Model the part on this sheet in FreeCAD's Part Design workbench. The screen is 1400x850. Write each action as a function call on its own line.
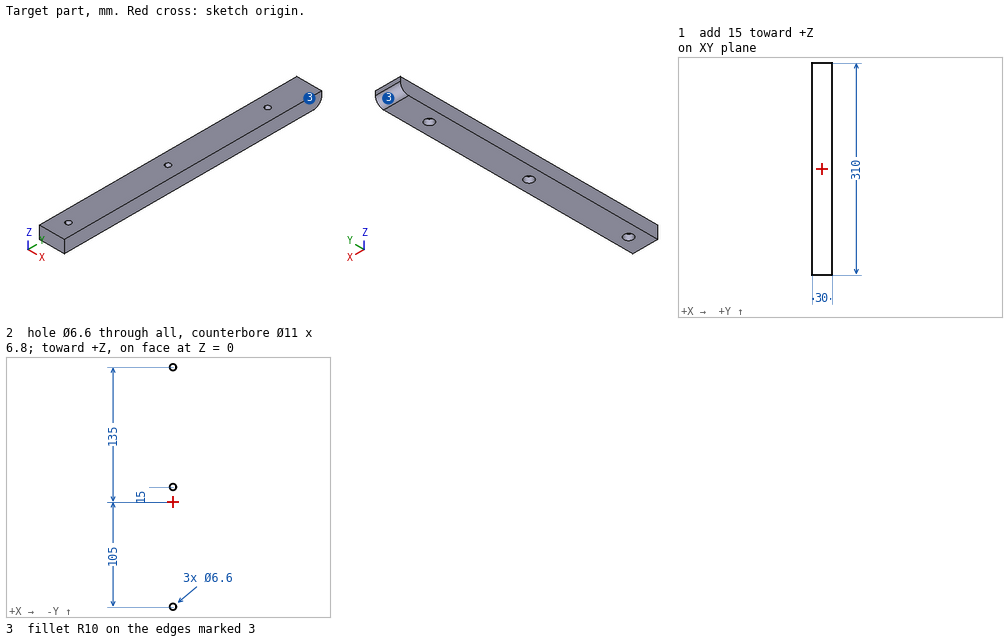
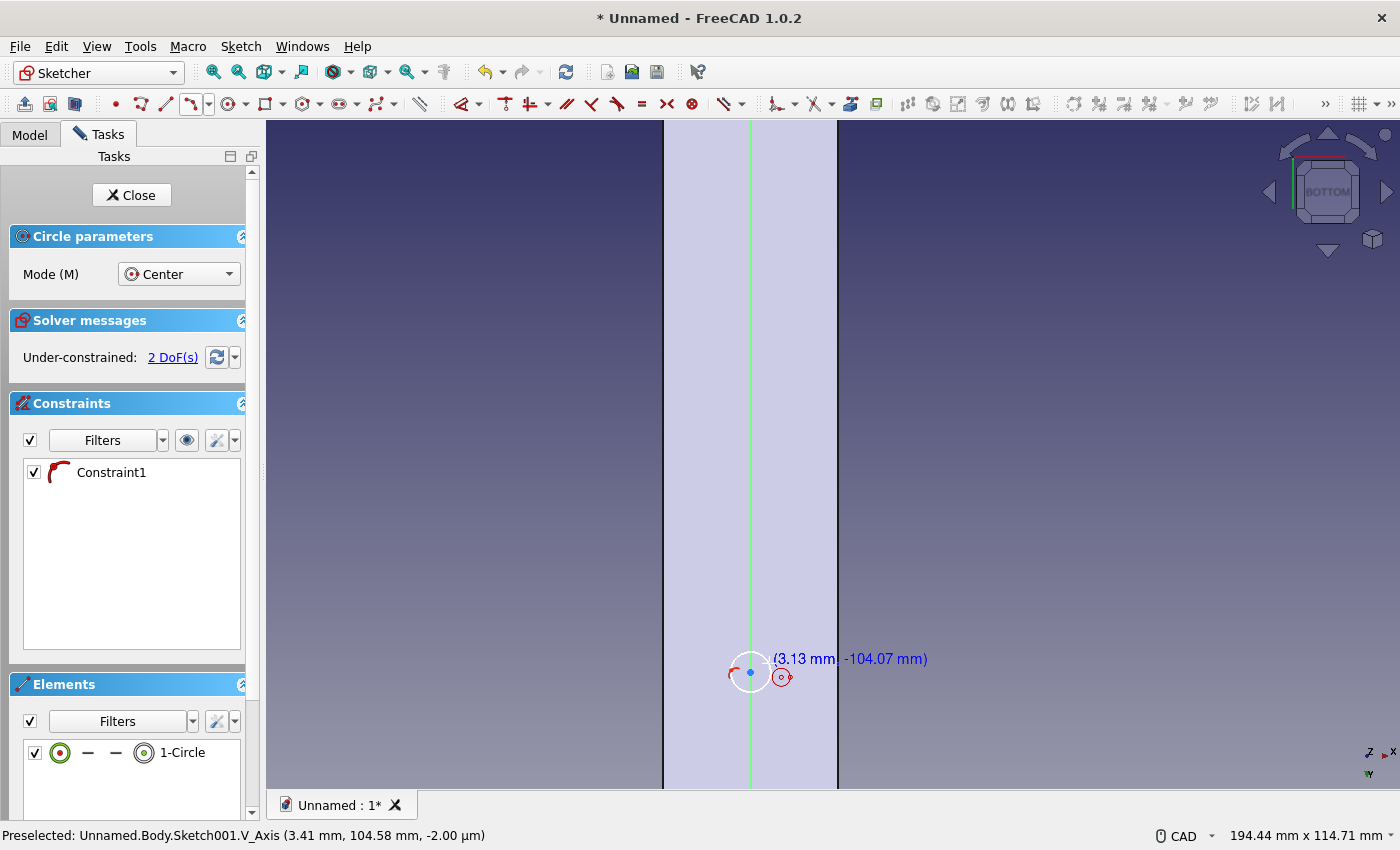
scroll(770, 664, down, 6)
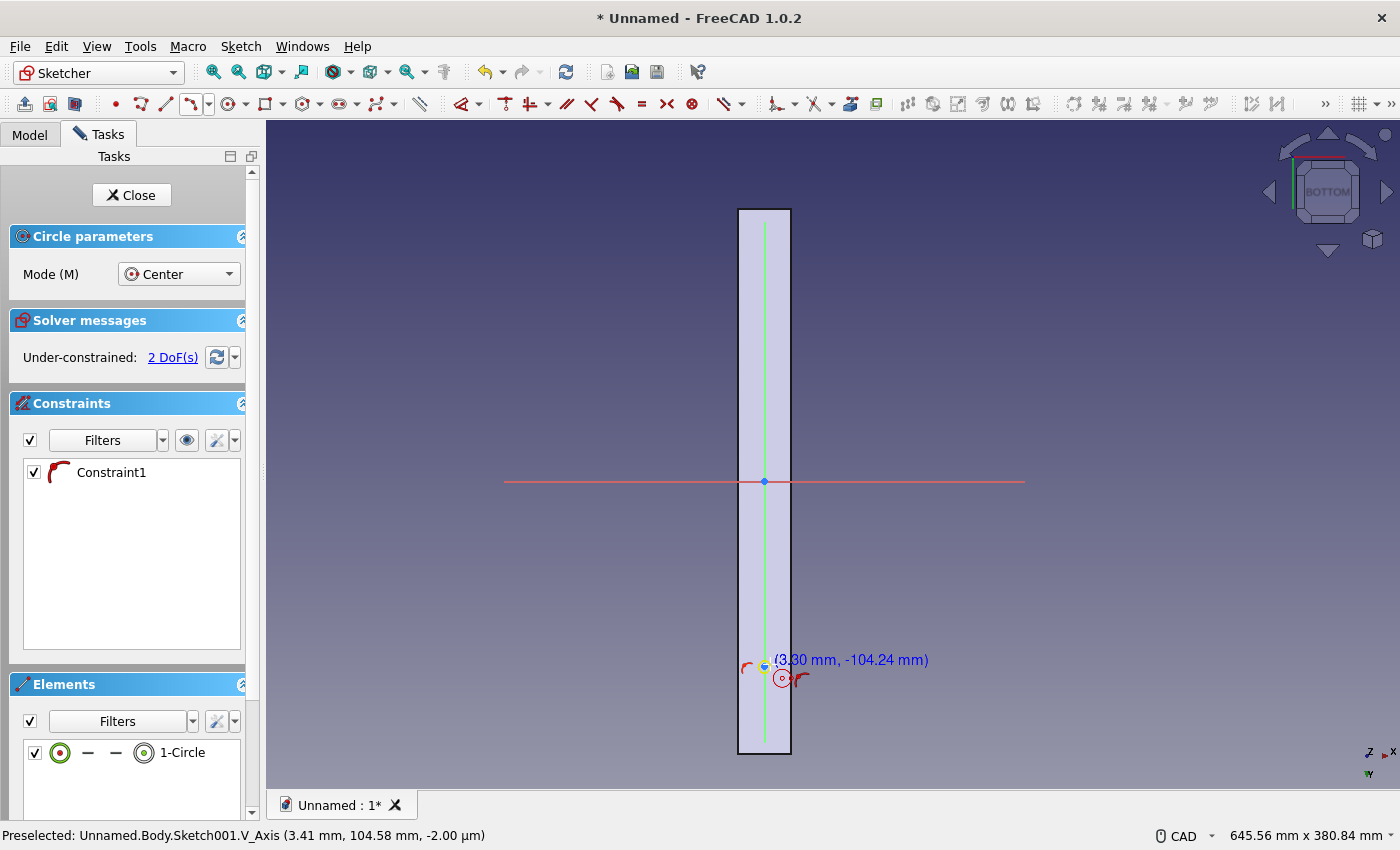
scroll(765, 455, up, 7)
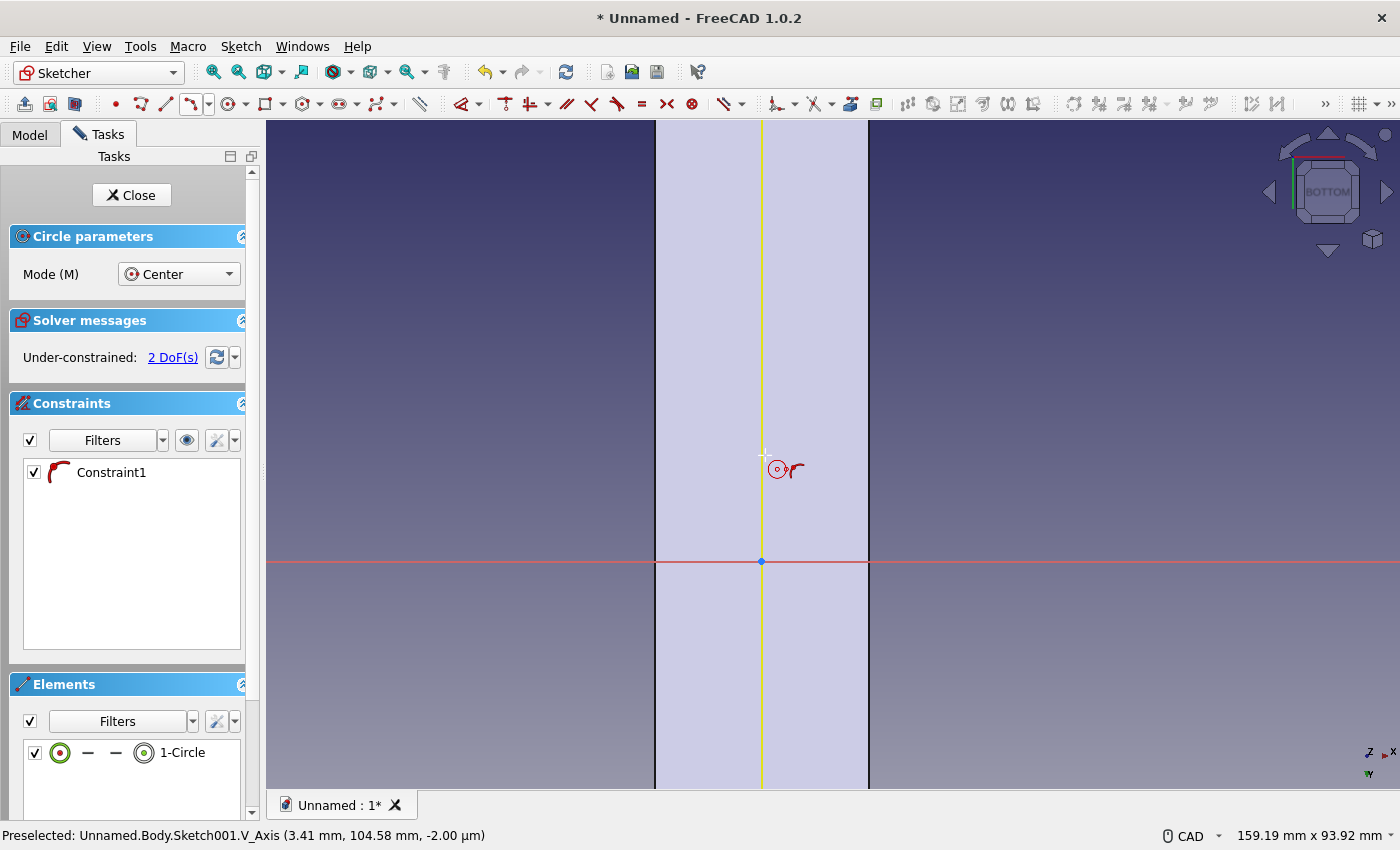
scroll(765, 454, down, 7)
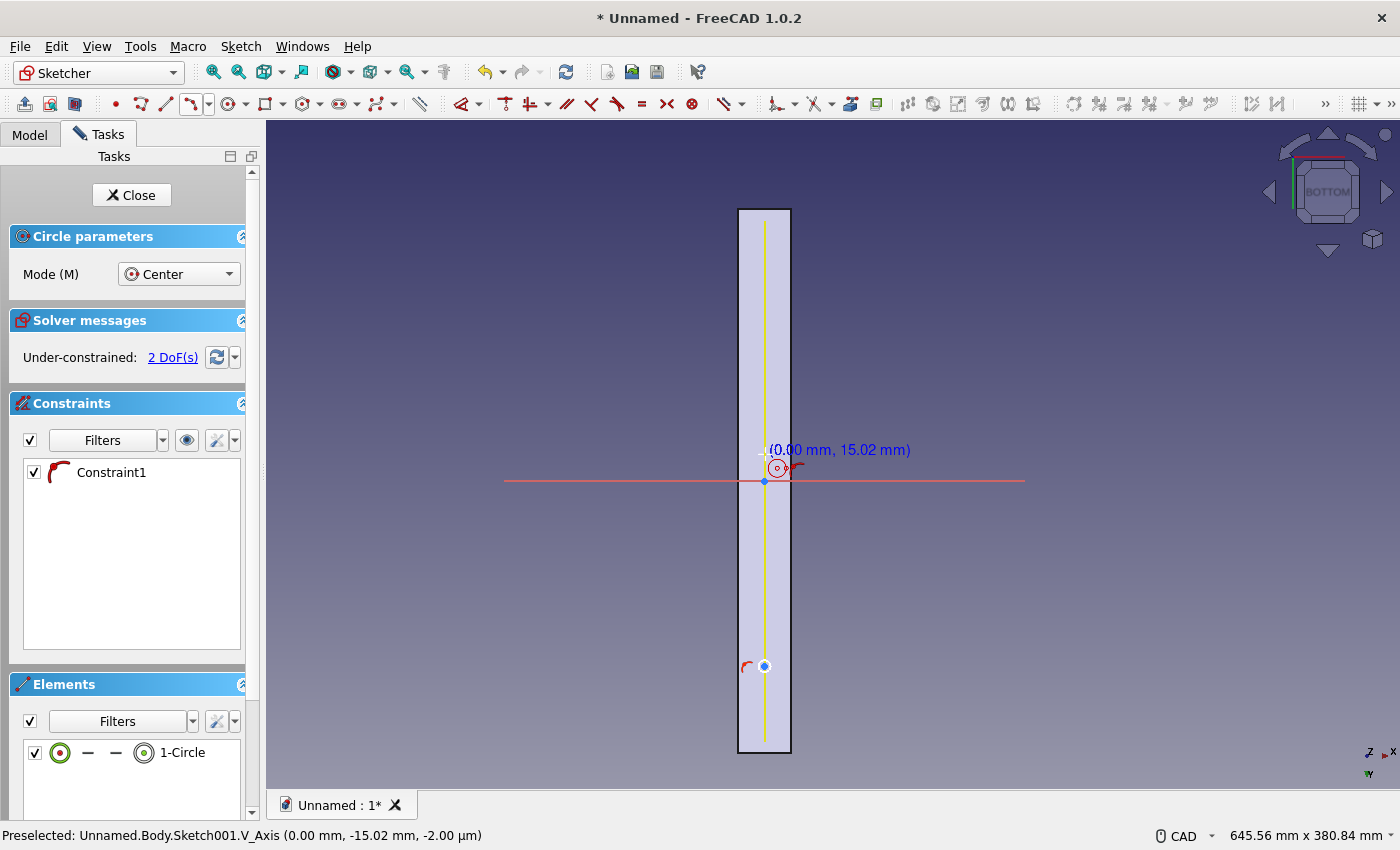
click(765, 455)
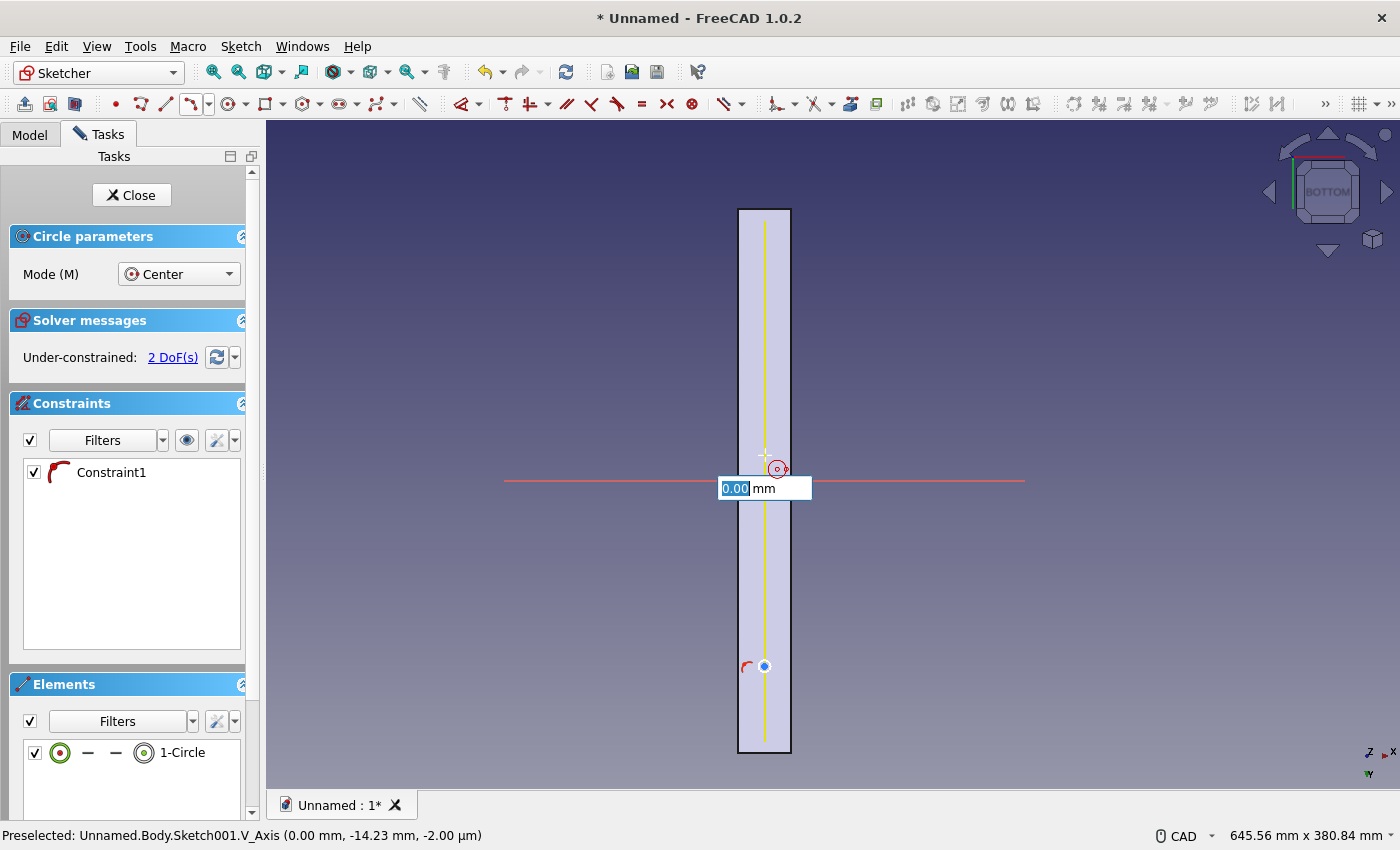
scroll(770, 453, up, 6)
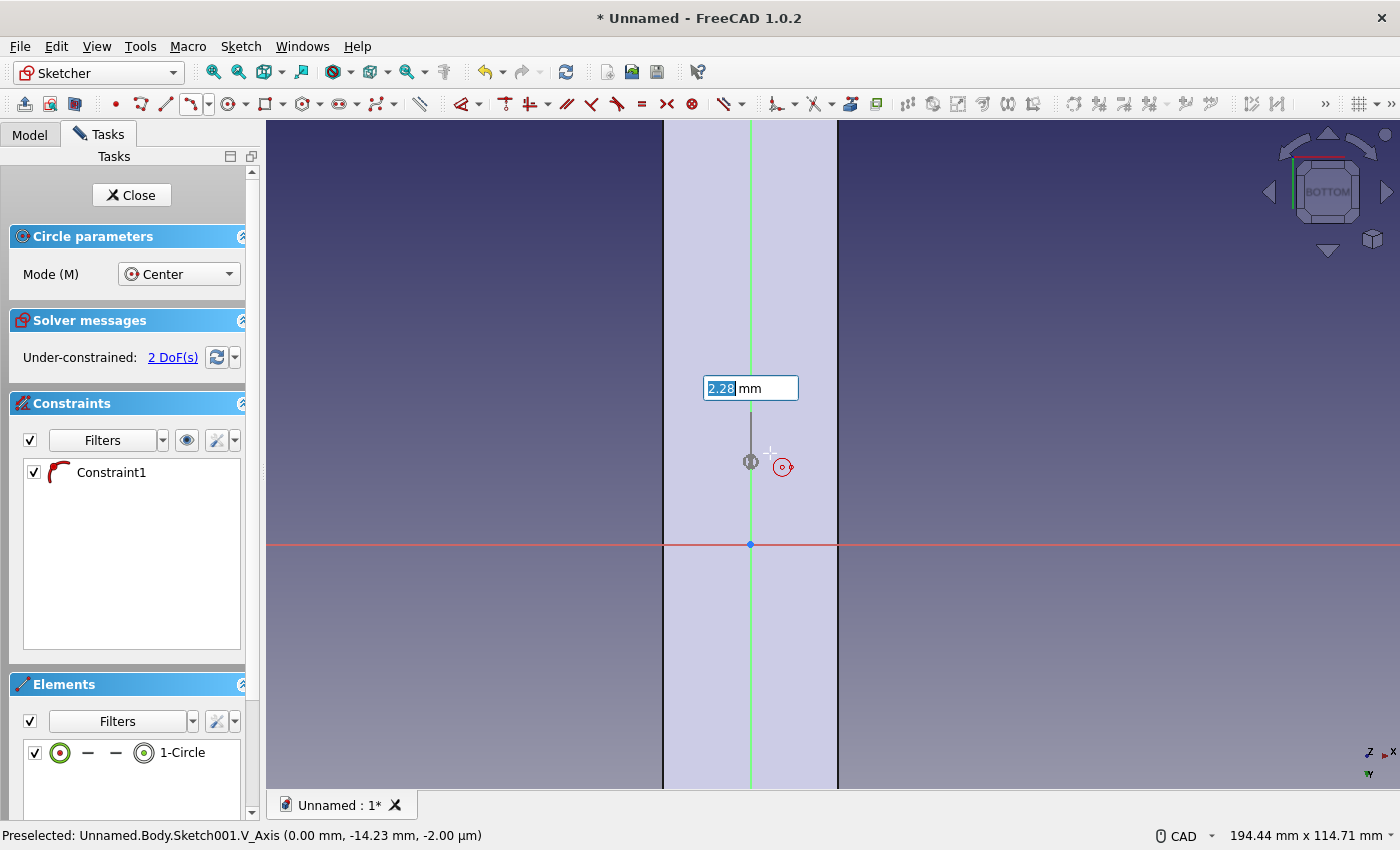
click(769, 451)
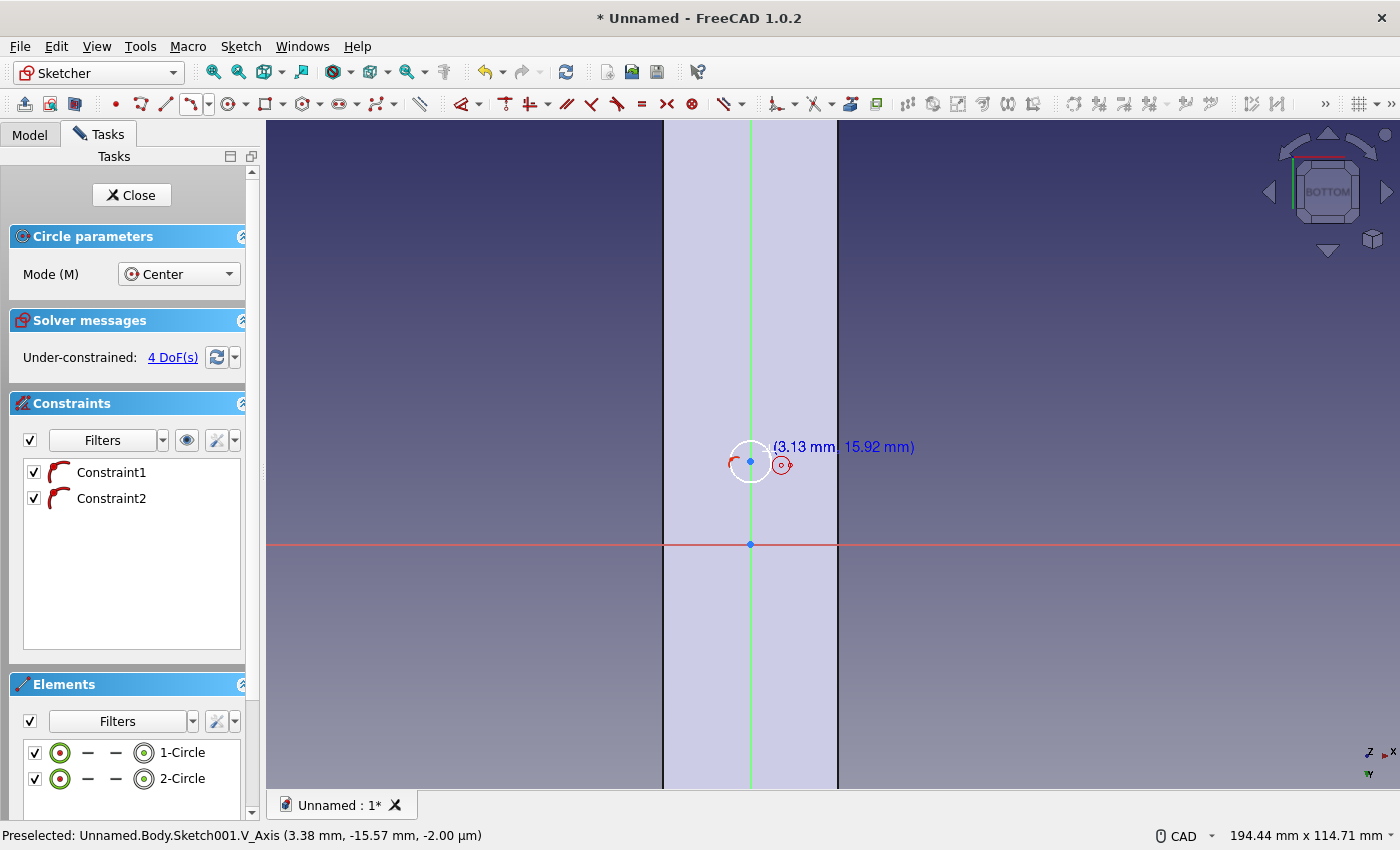
scroll(770, 453, down, 6)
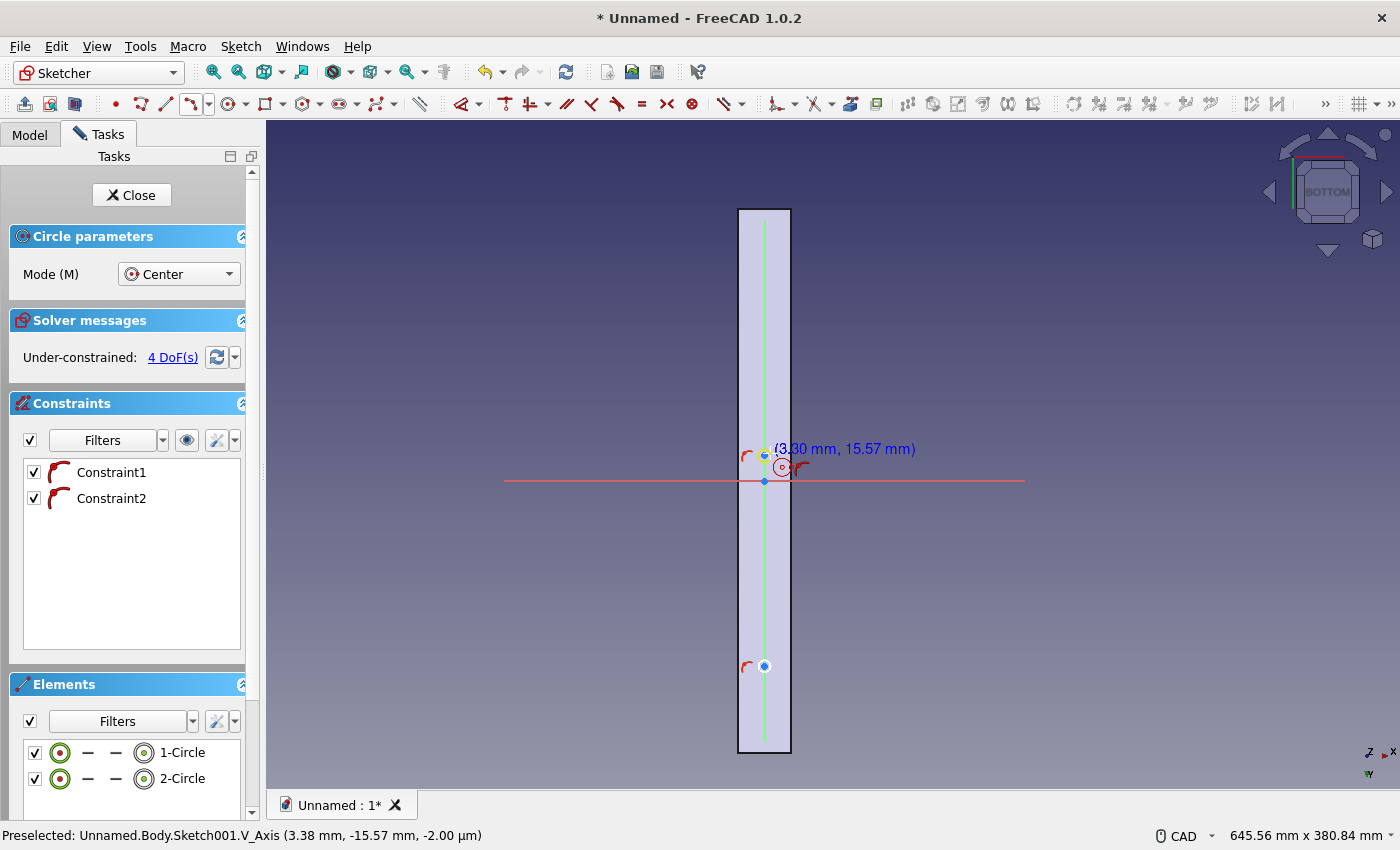
scroll(765, 244, up, 7)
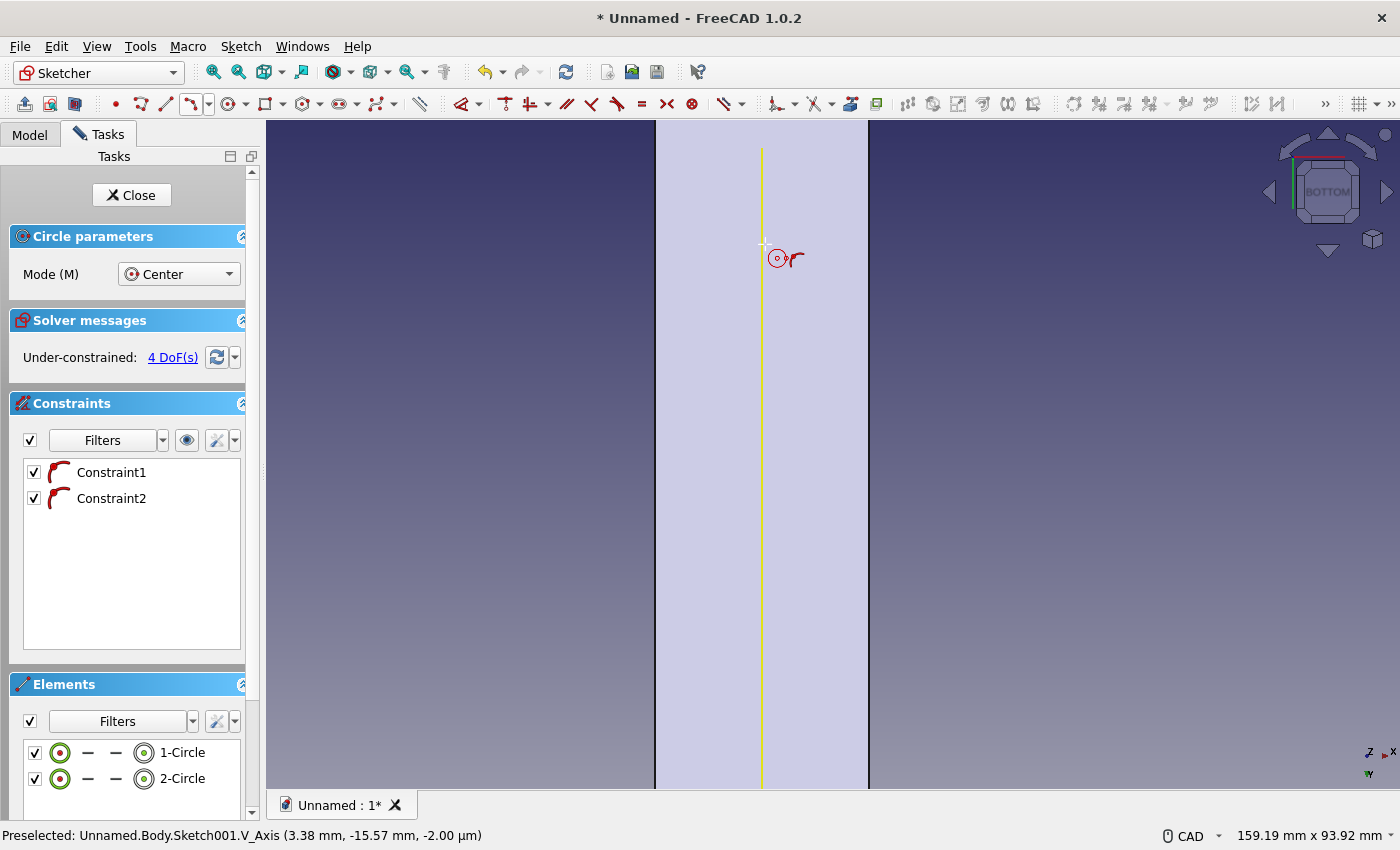
scroll(765, 244, down, 7)